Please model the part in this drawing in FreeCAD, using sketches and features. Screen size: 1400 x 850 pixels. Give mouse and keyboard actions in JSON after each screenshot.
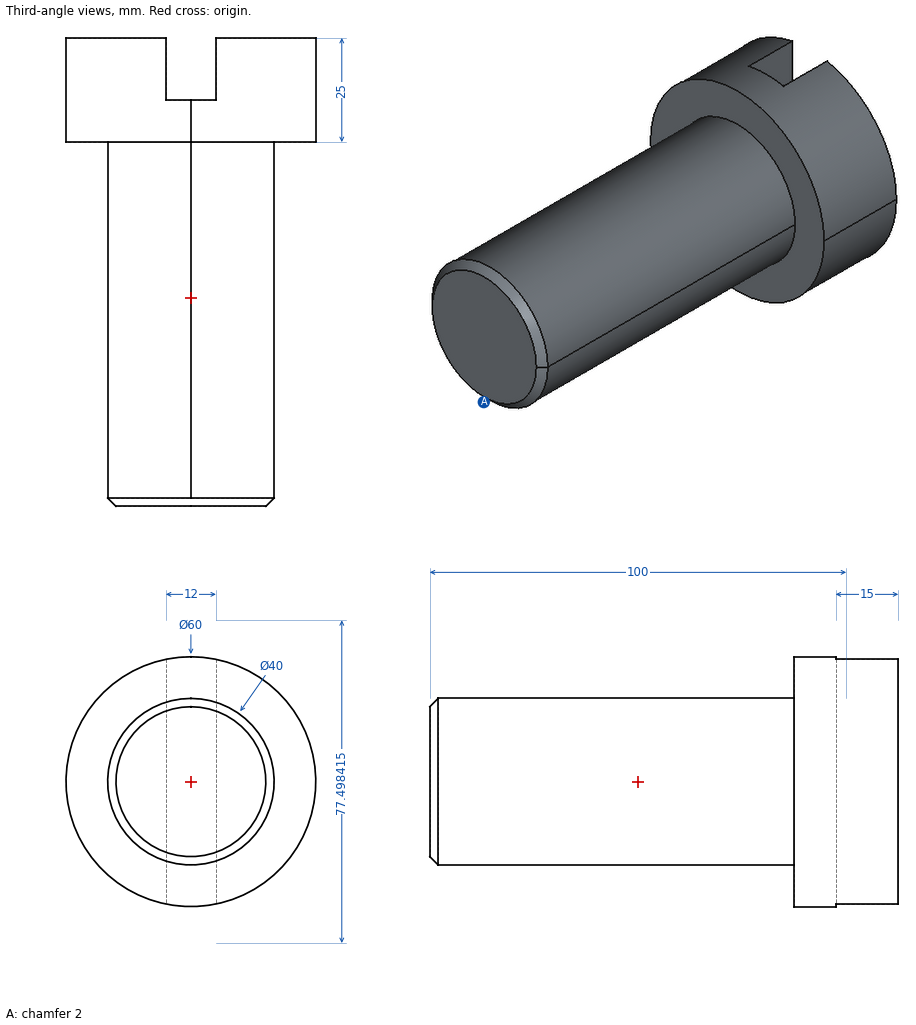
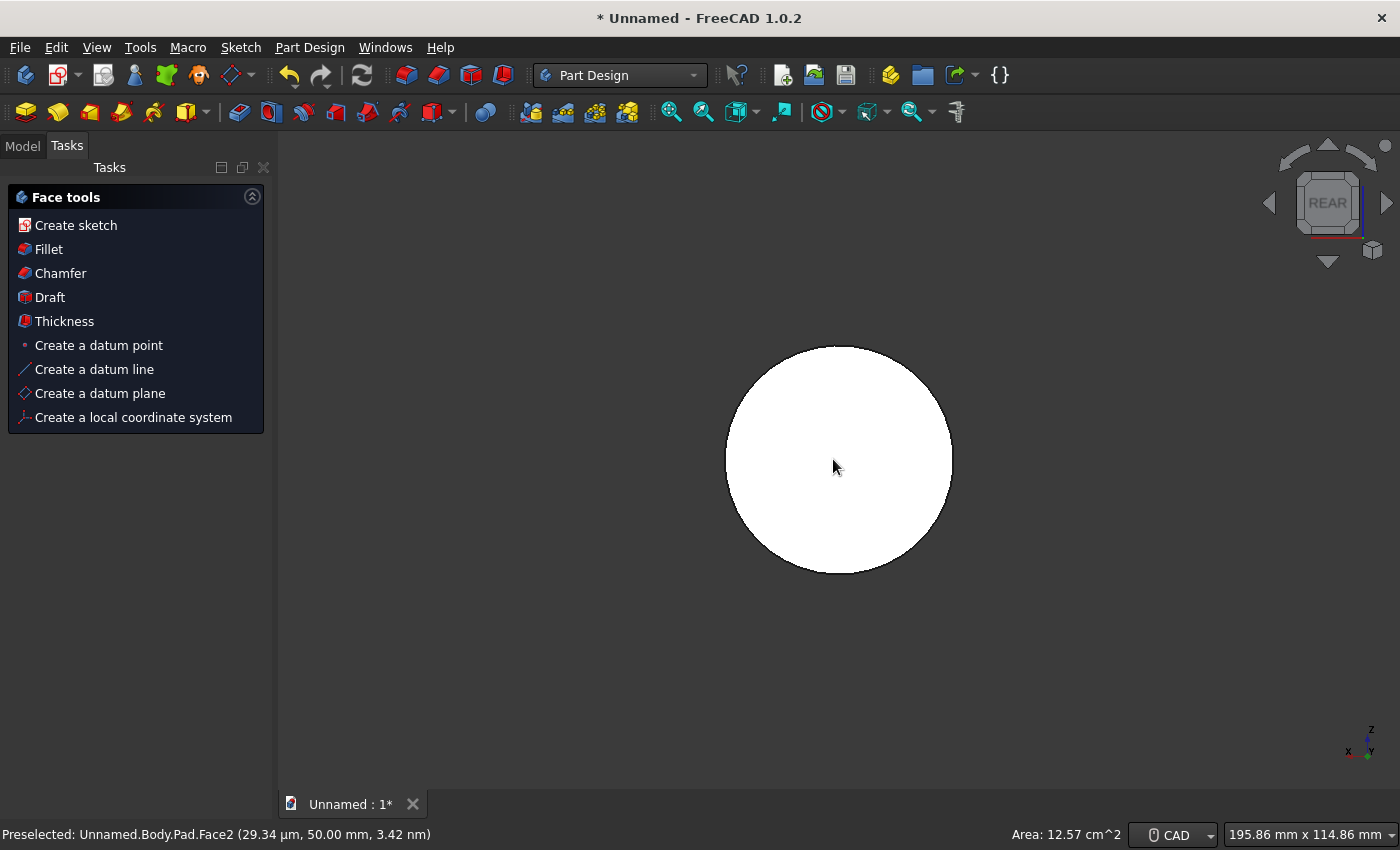
{"action": "left_click", "coordinate": [58, 76]}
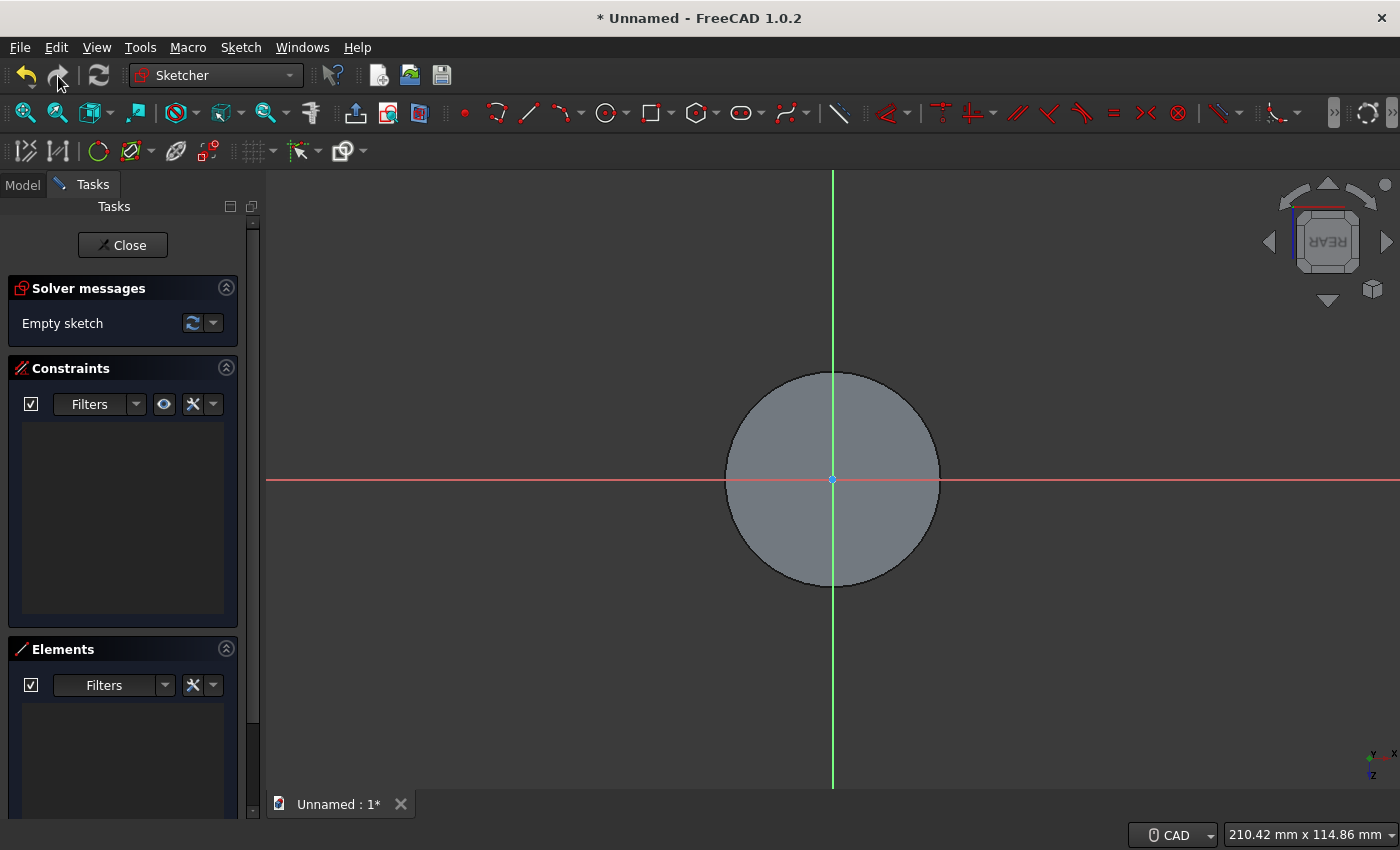
{"action": "left_click", "coordinate": [606, 114]}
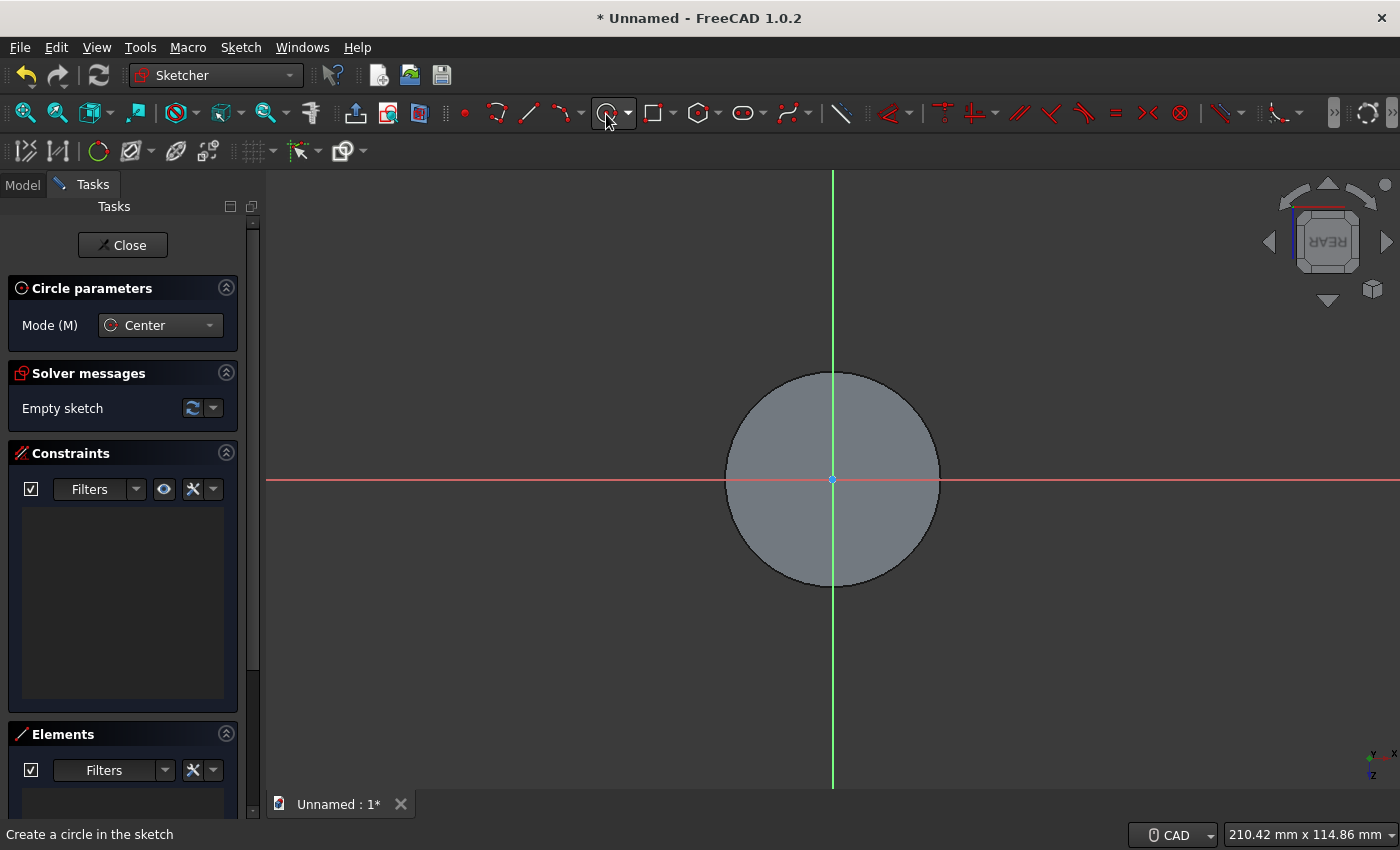
{"action": "left_click", "coordinate": [833, 479]}
{"action": "mouse_move", "coordinate": [947, 365]}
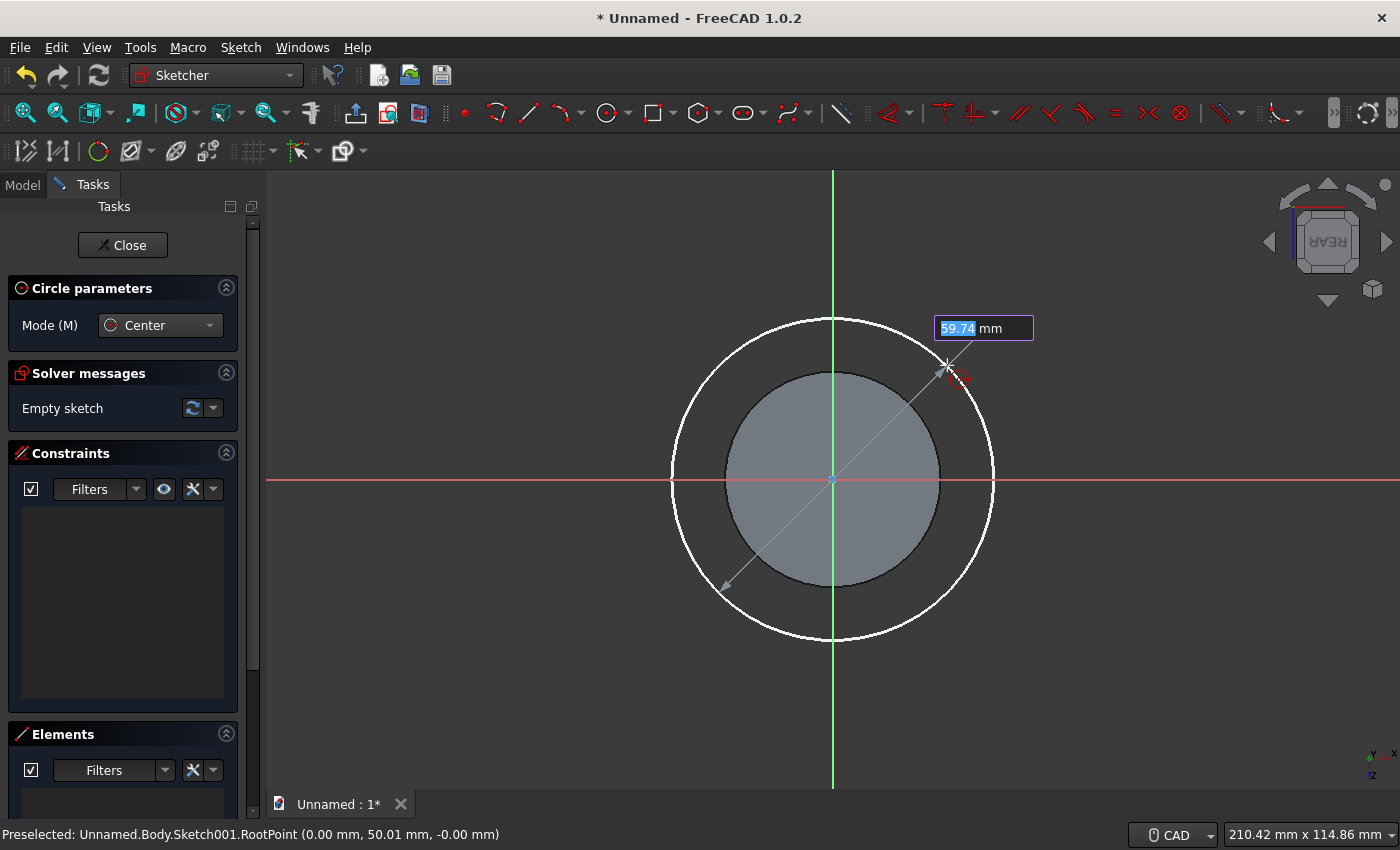
{"action": "type", "text": "60"}
{"action": "key", "text": "Return"}
{"action": "key", "text": "Escape"}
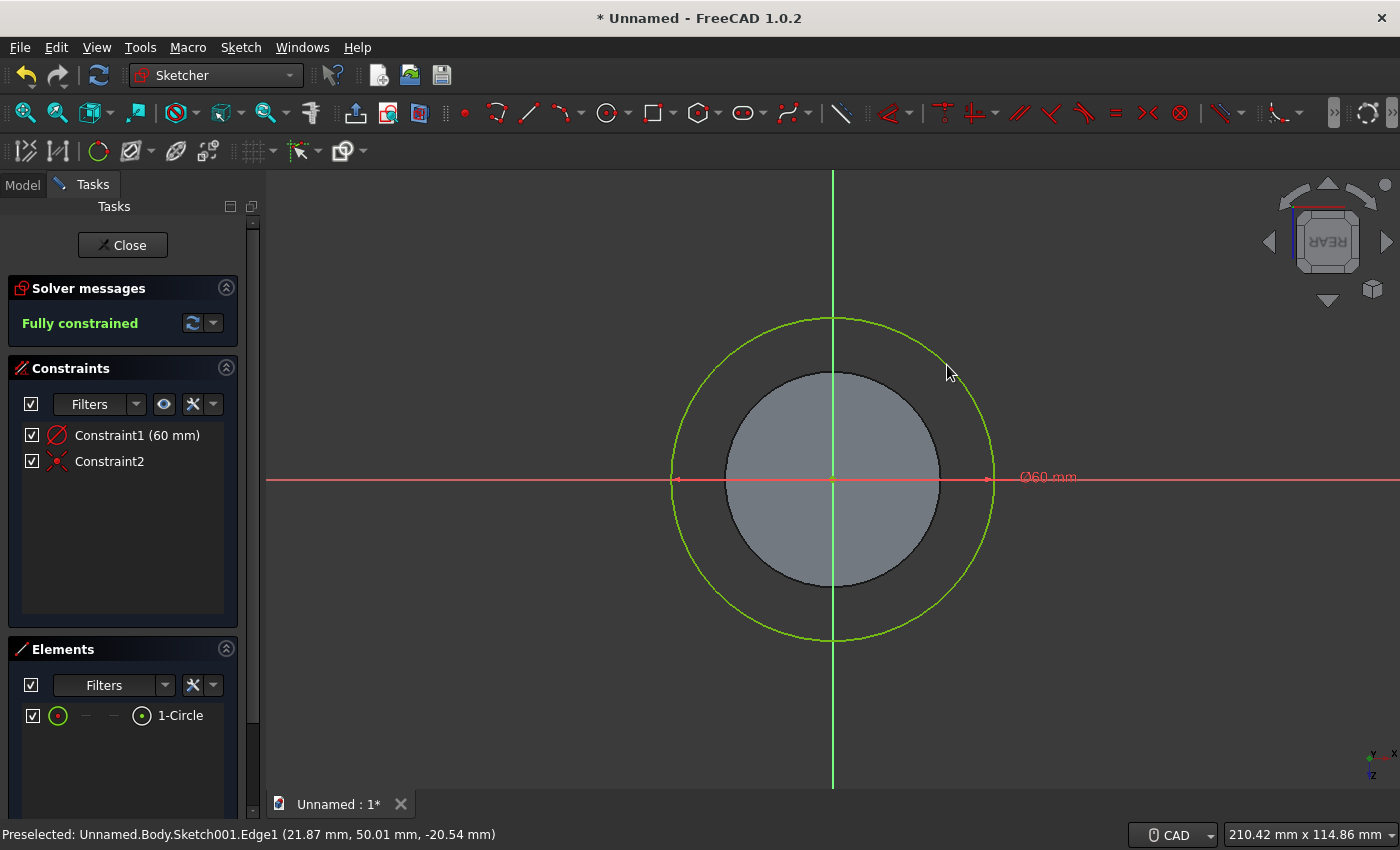
{"action": "left_click", "coordinate": [123, 245]}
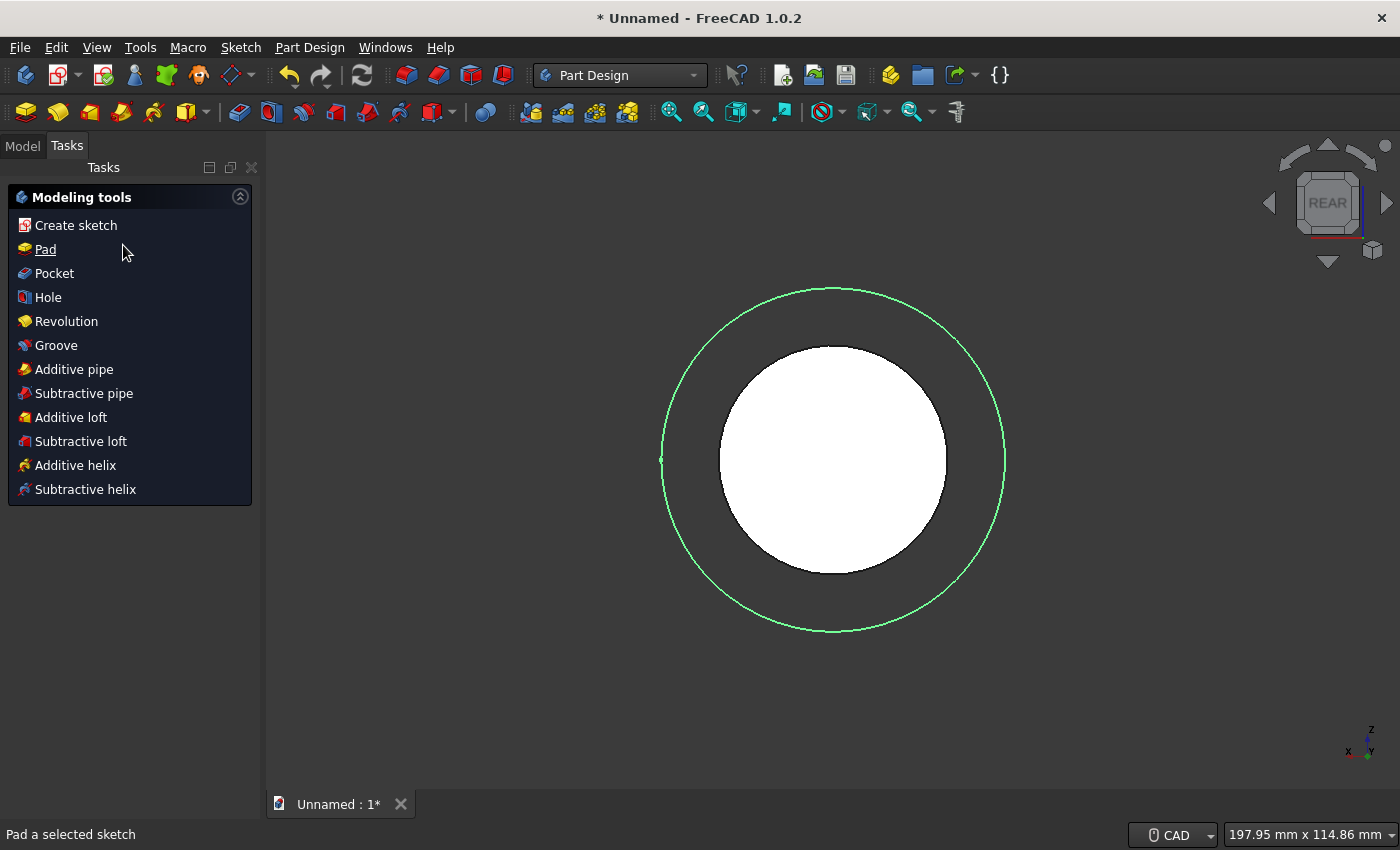
{"action": "left_click", "coordinate": [26, 112]}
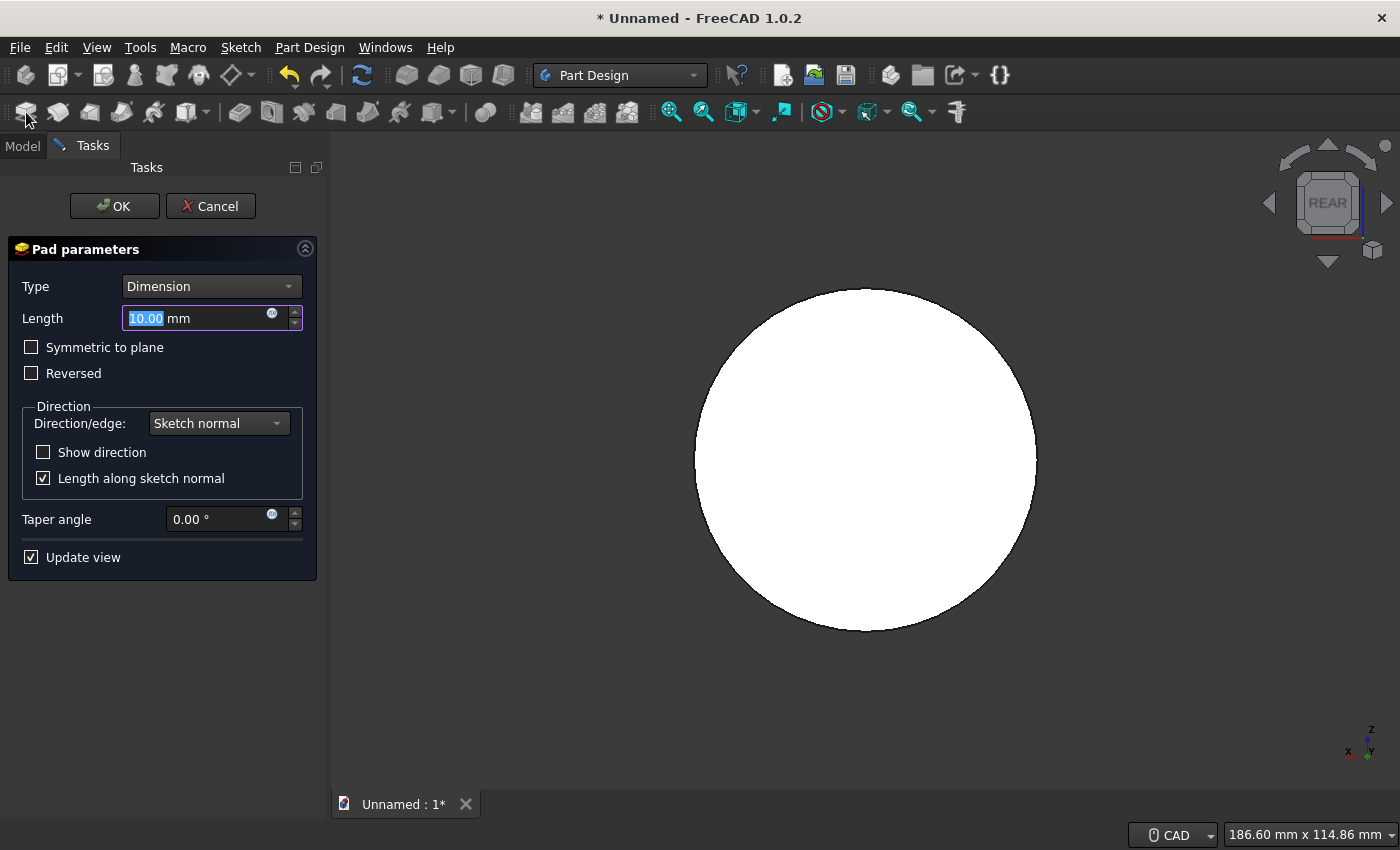
{"action": "type", "text": "25"}
{"action": "key", "text": "Tab"}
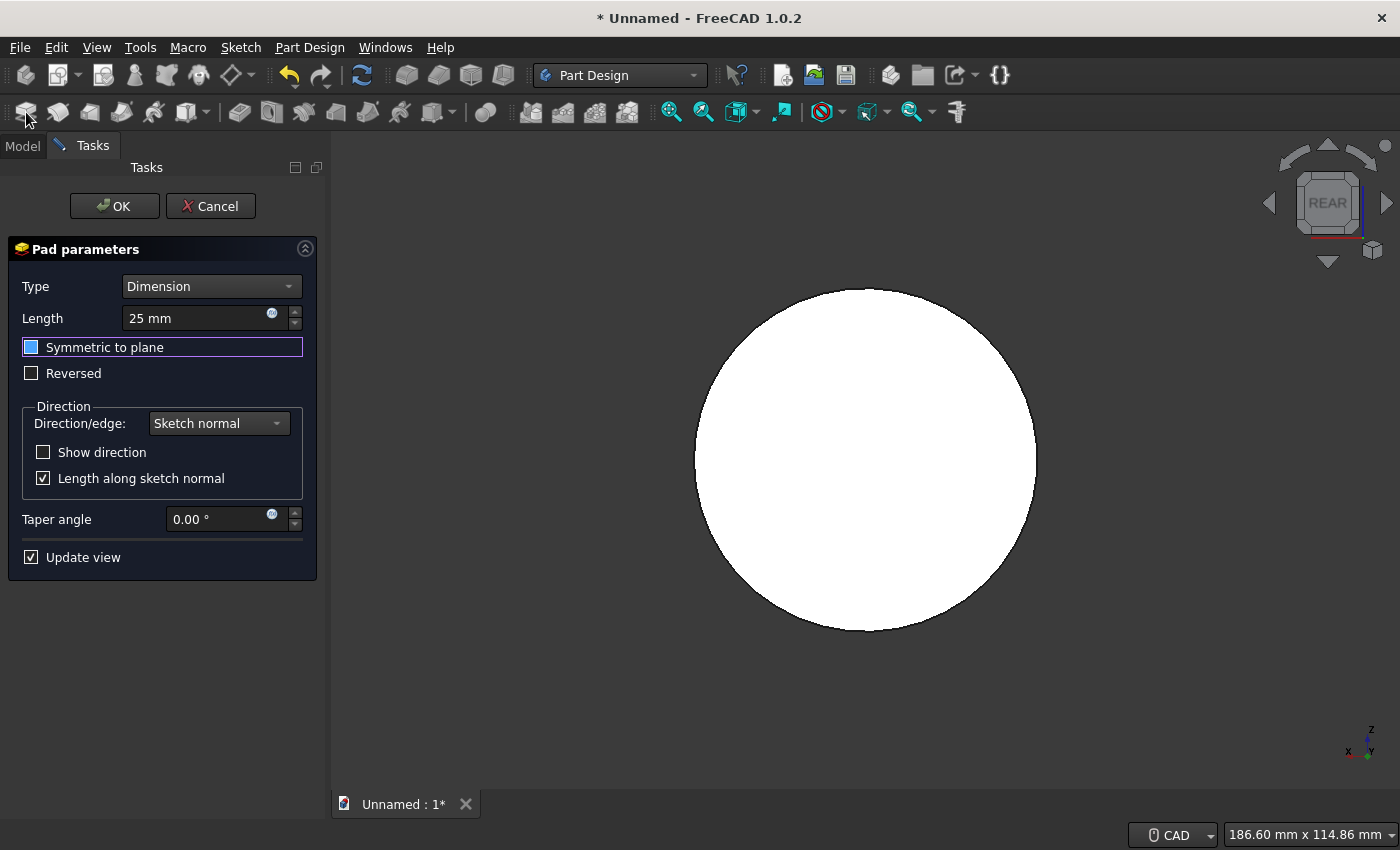
{"action": "left_click", "coordinate": [30, 347]}